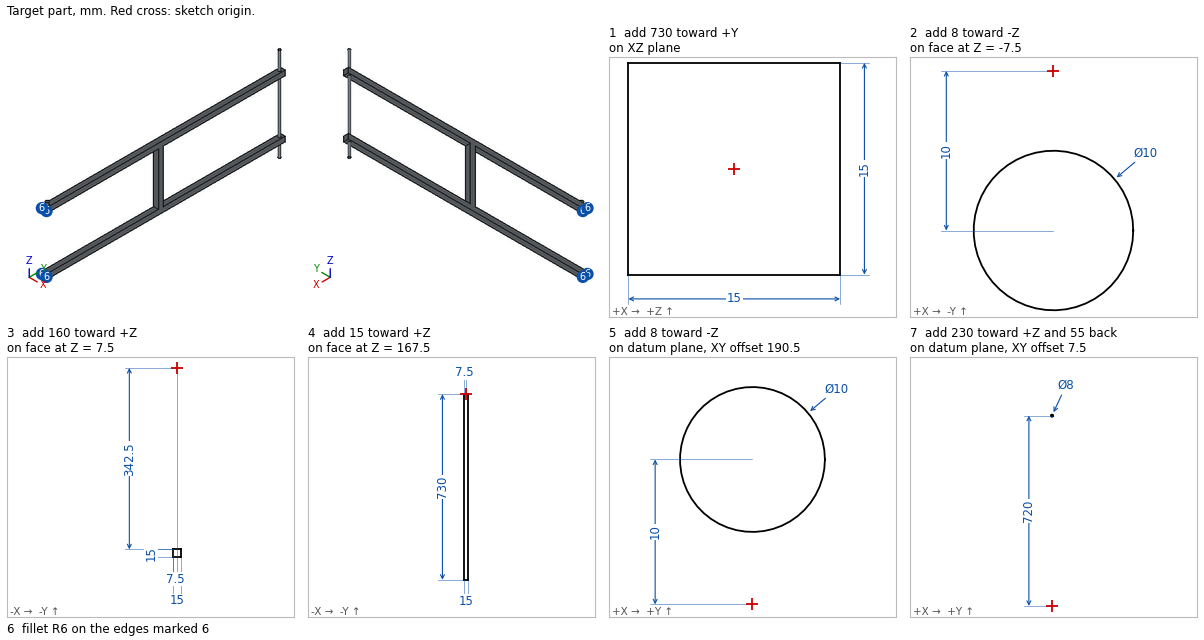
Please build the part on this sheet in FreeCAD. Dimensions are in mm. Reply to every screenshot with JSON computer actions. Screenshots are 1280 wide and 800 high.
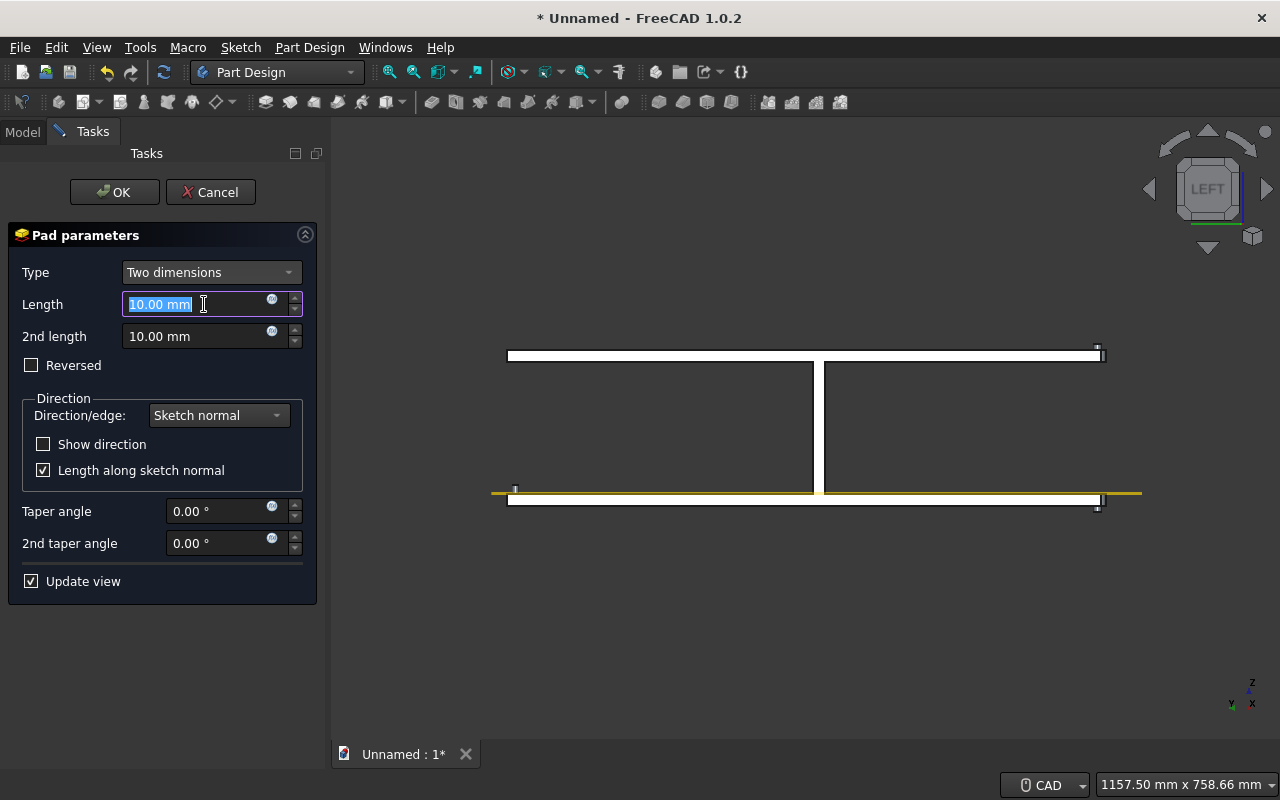
{"action": "type", "text": "230"}
{"action": "key", "text": "Tab"}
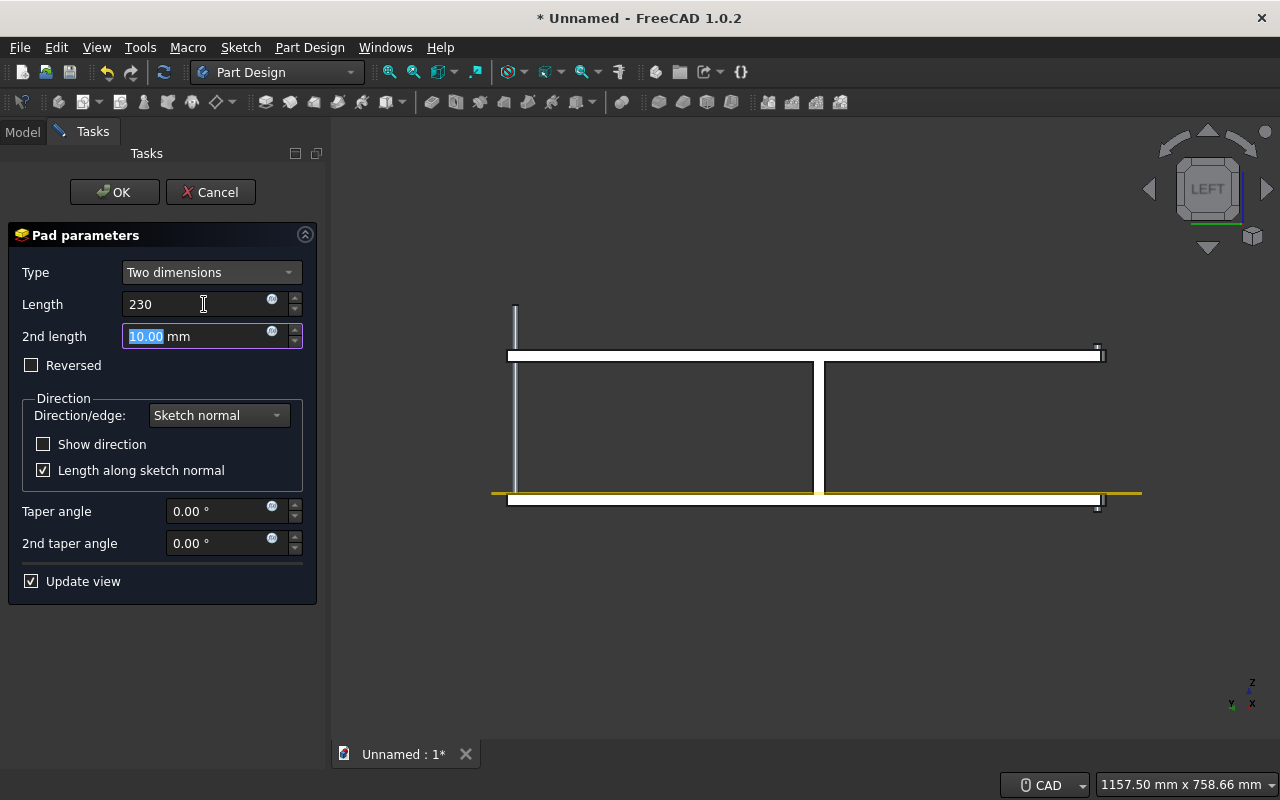
{"action": "type", "text": "55"}
{"action": "key", "text": "Tab"}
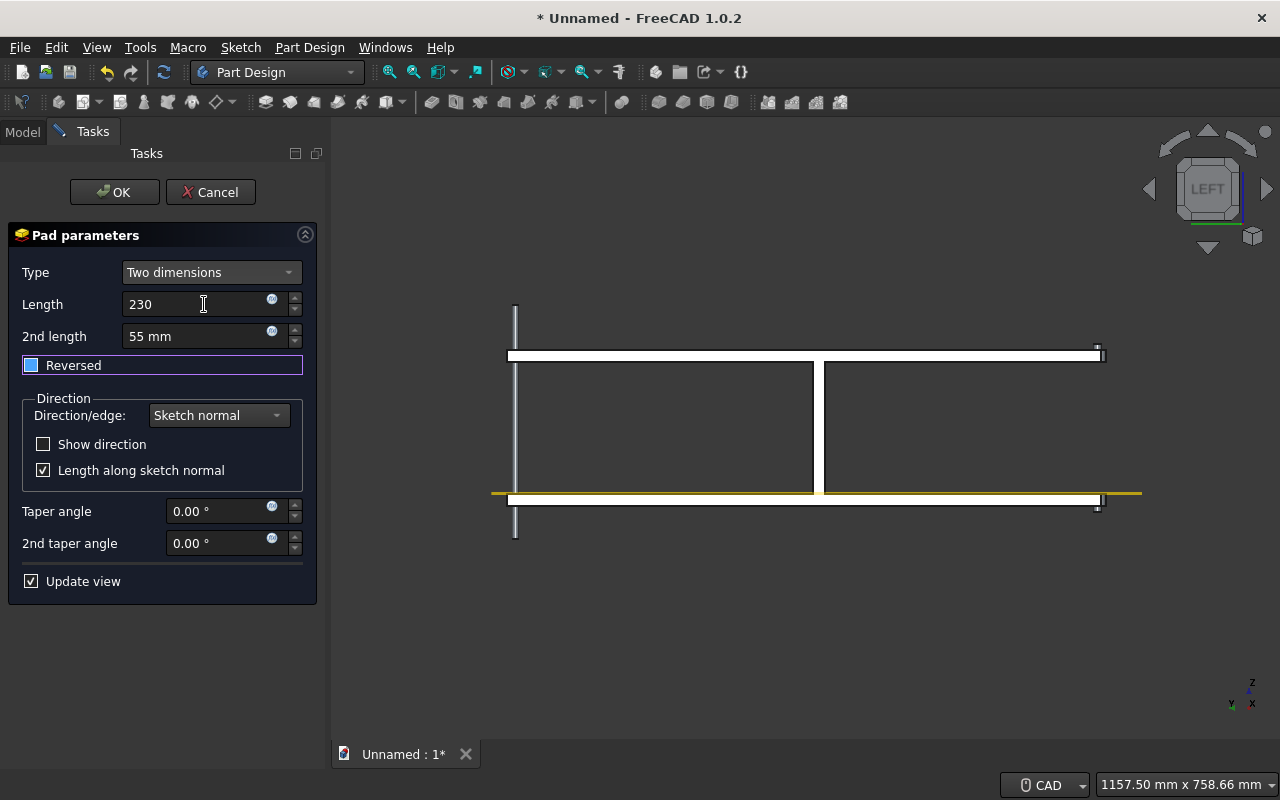
{"action": "left_click", "coordinate": [115, 192]}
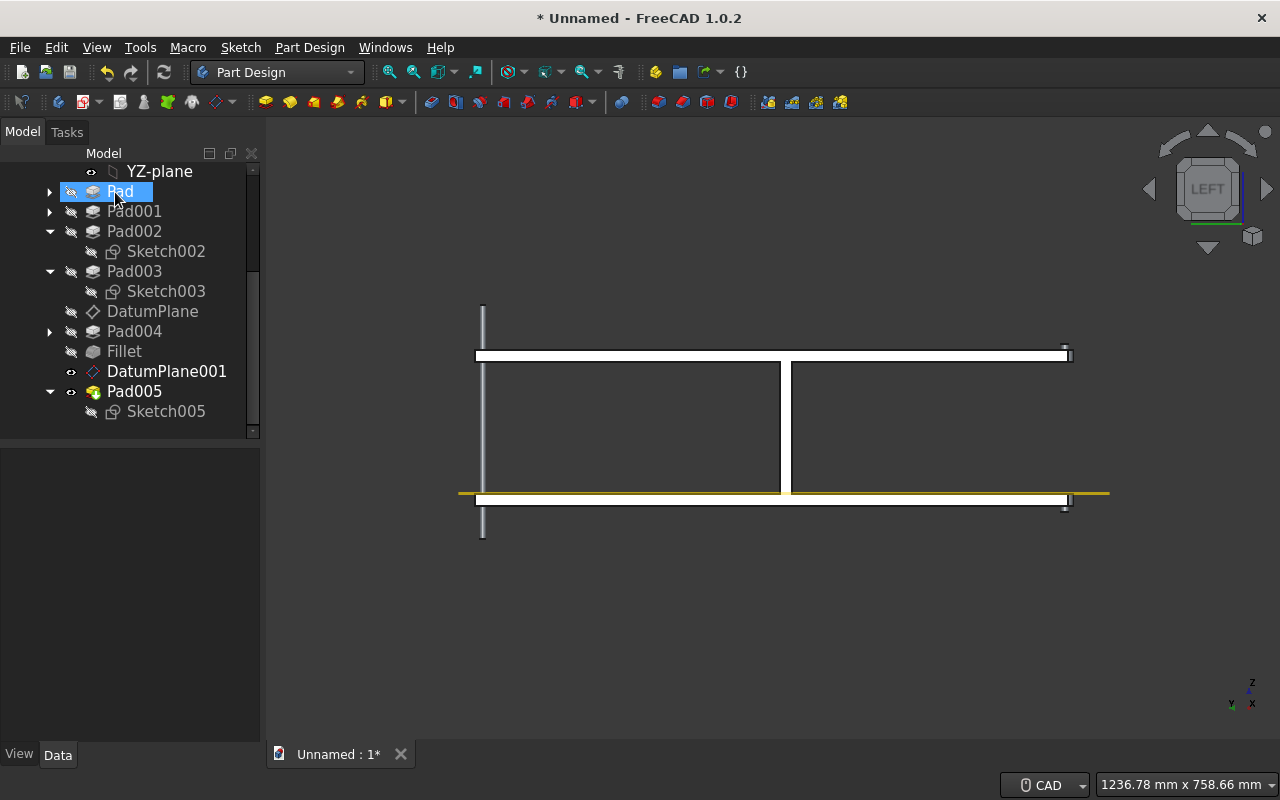
{"action": "left_click", "coordinate": [116, 372]}
{"action": "key", "text": "space"}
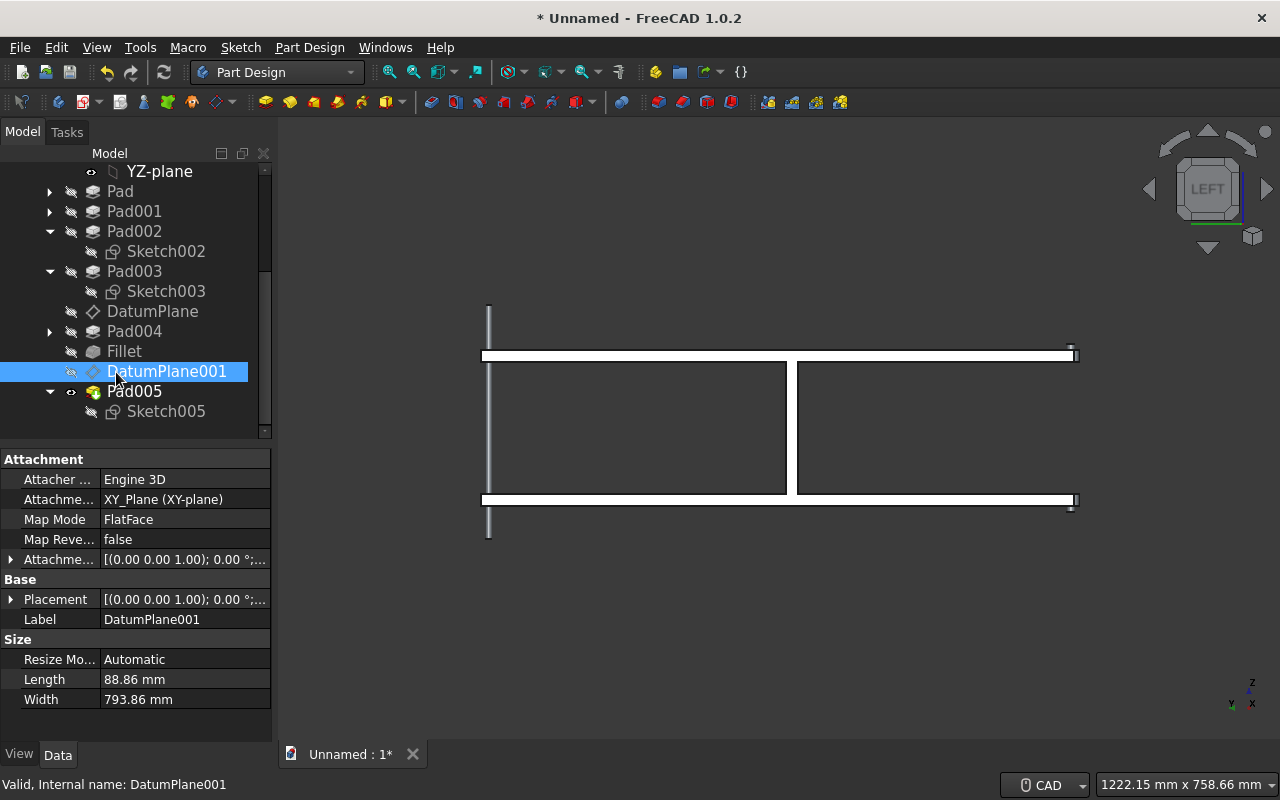
{"action": "key", "text": "0"}